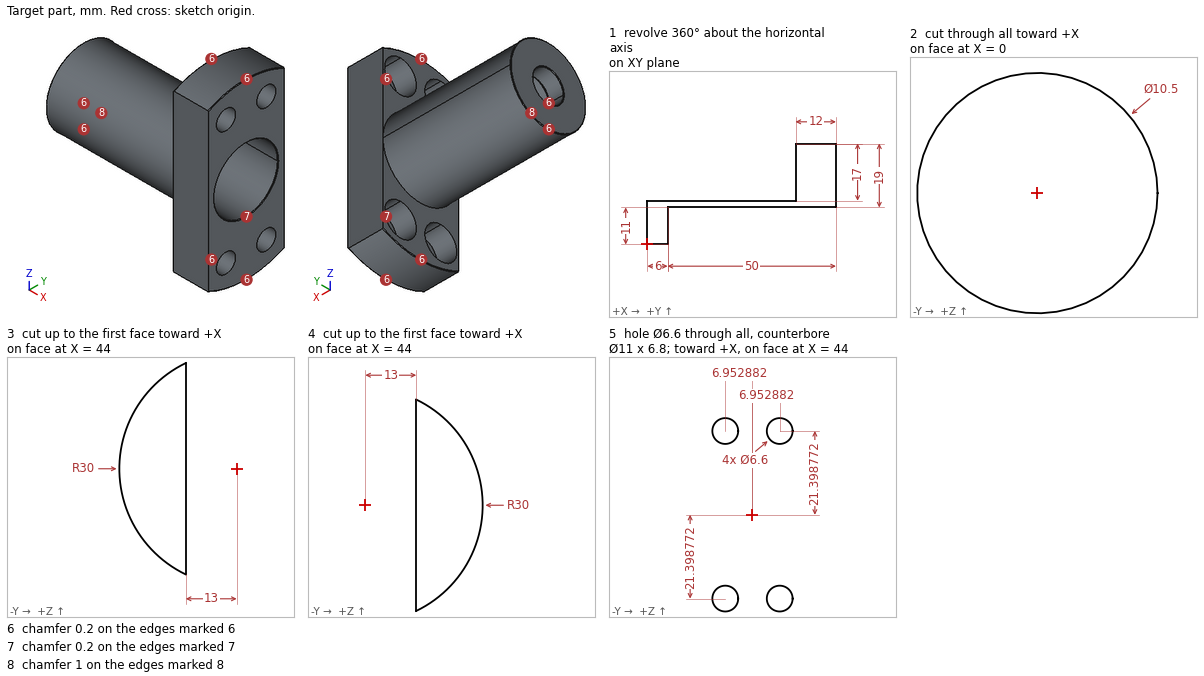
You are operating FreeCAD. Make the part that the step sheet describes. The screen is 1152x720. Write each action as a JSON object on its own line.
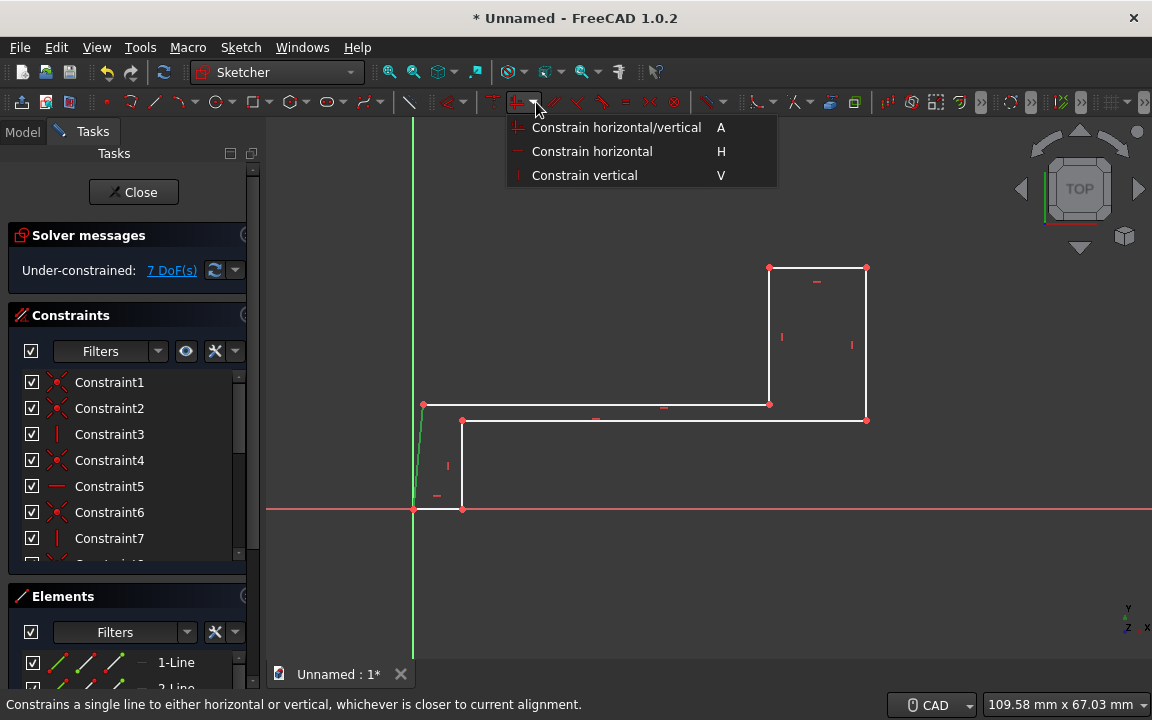
{"action": "left_click", "coordinate": [642, 175]}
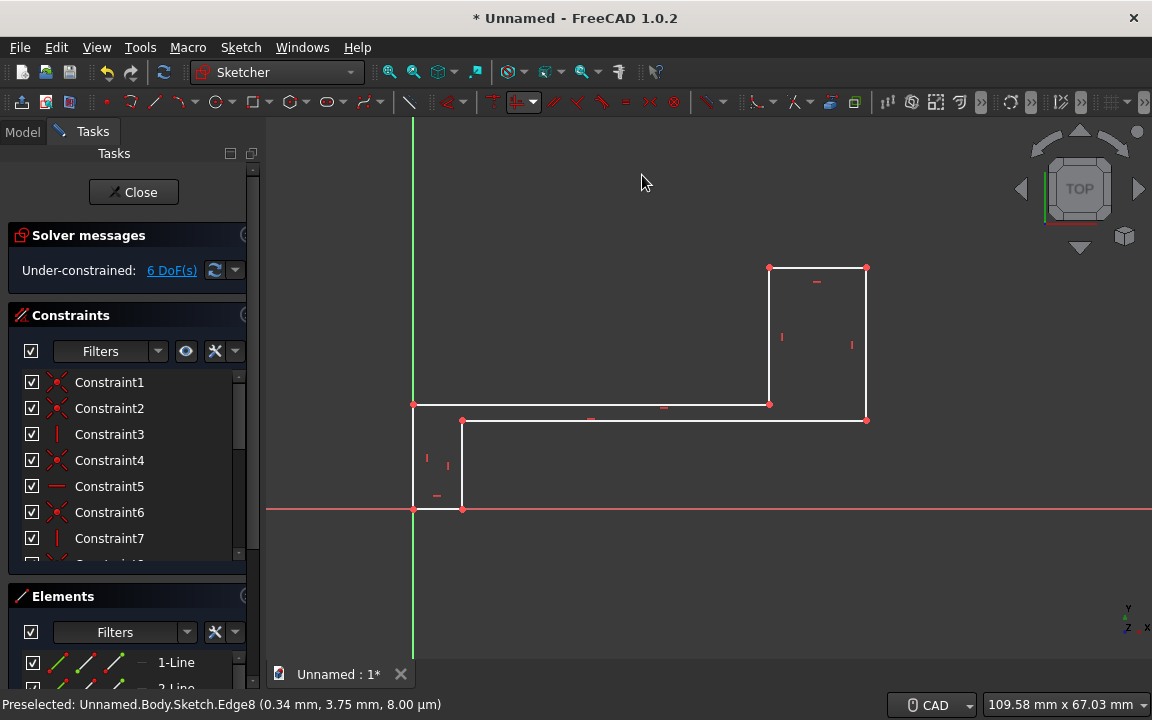
{"action": "left_click", "coordinate": [428, 509]}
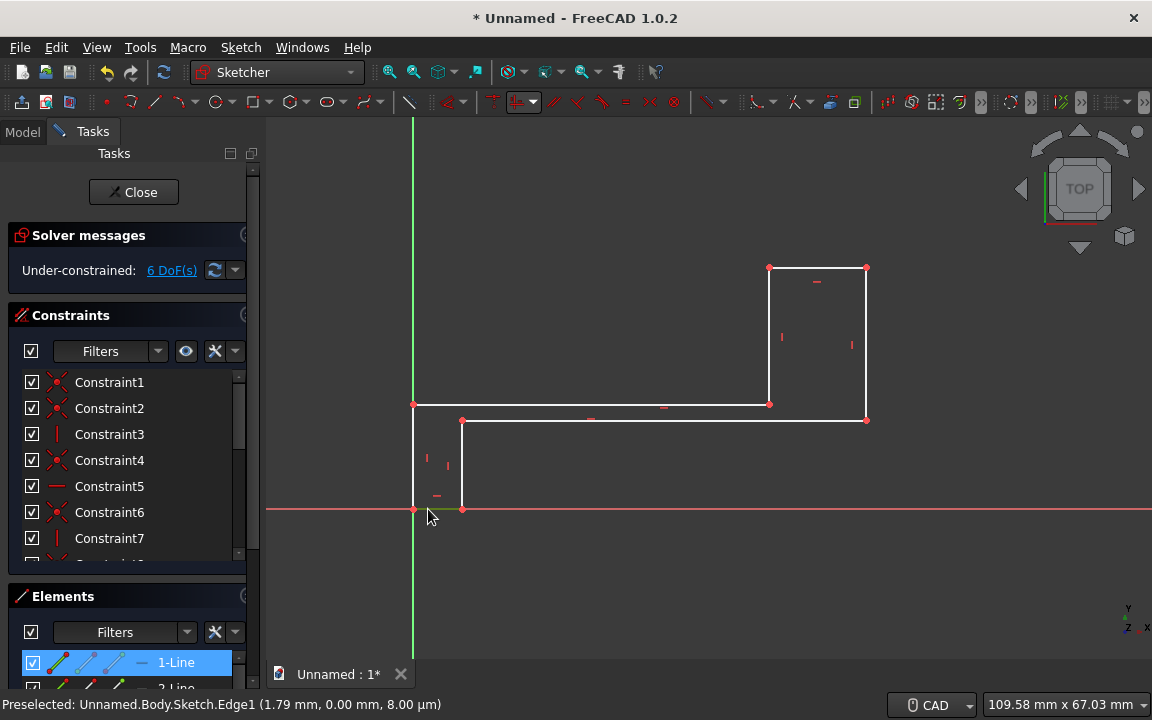
{"action": "key", "text": "l"}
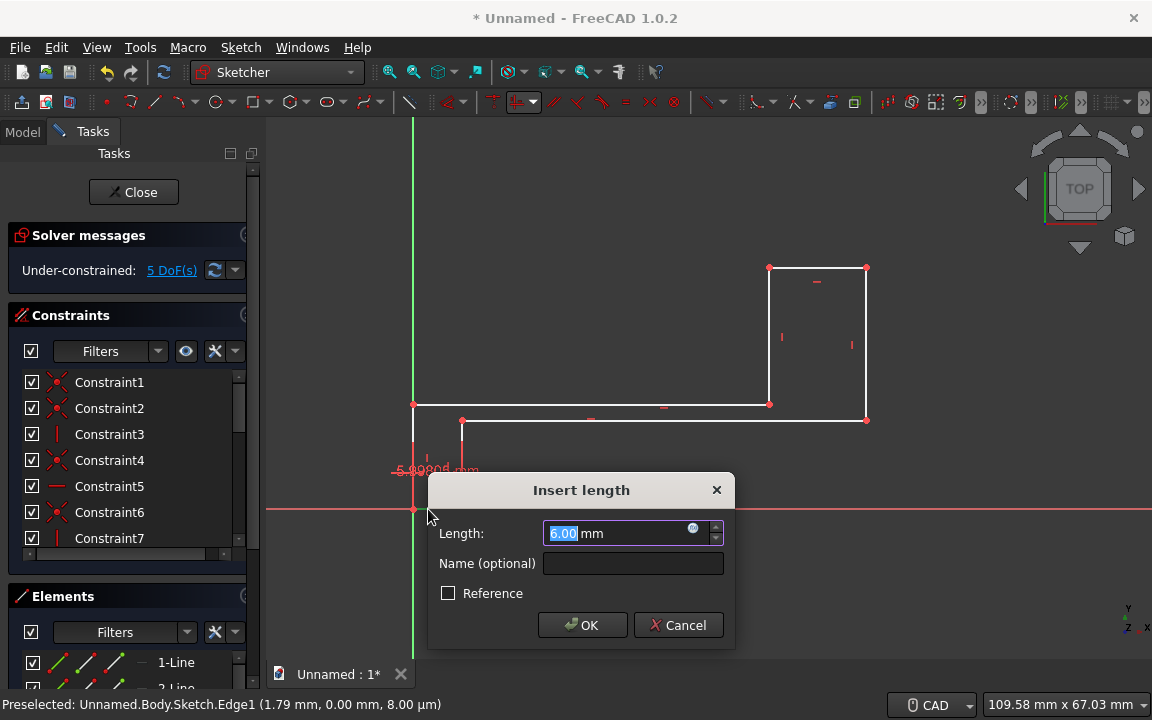
{"action": "type", "text": "6"}
{"action": "key", "text": "Return"}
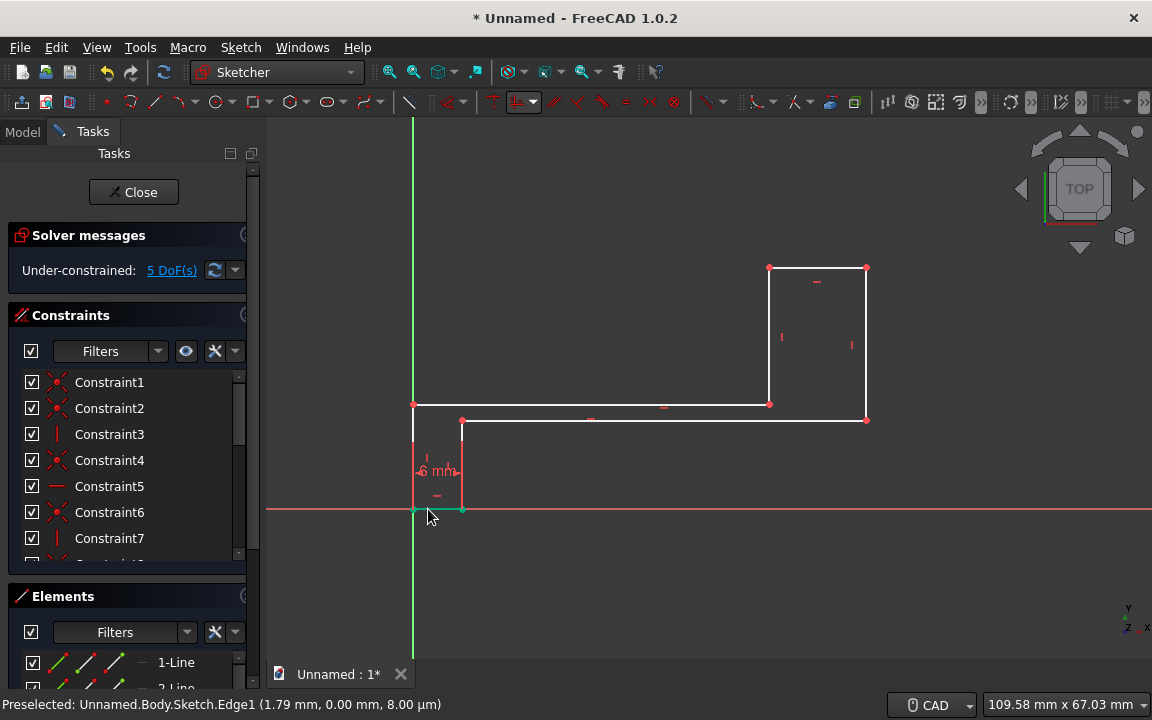
{"action": "left_click", "coordinate": [462, 483]}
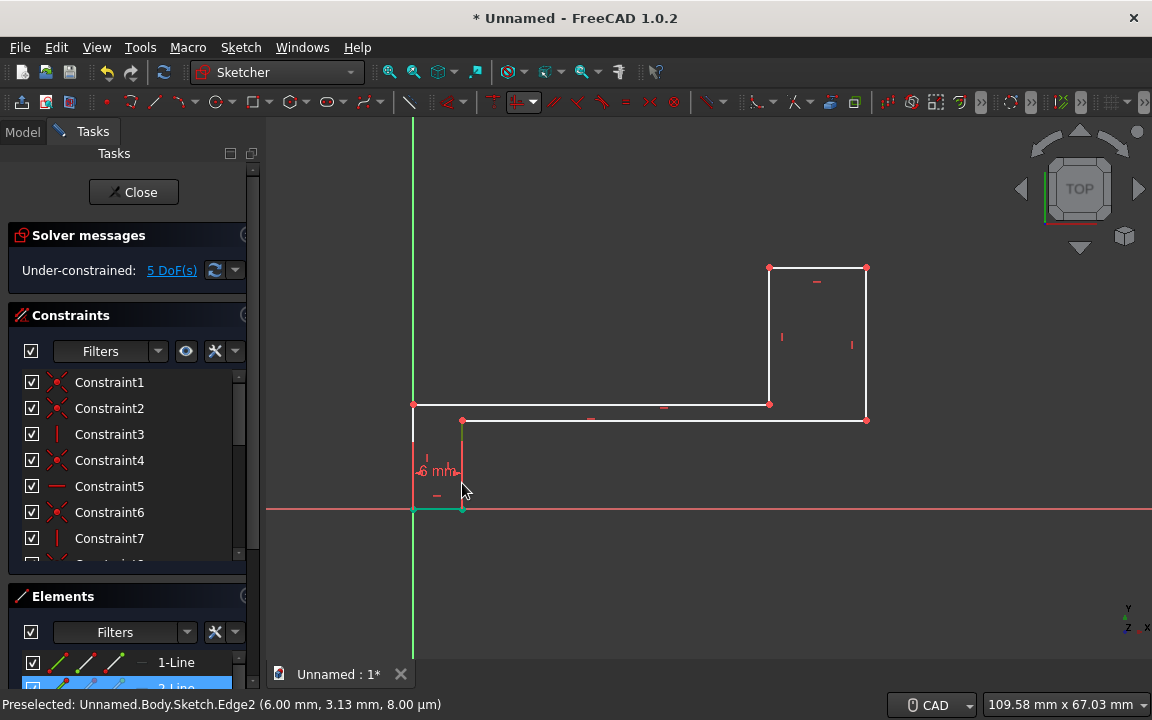
{"action": "key", "text": "i"}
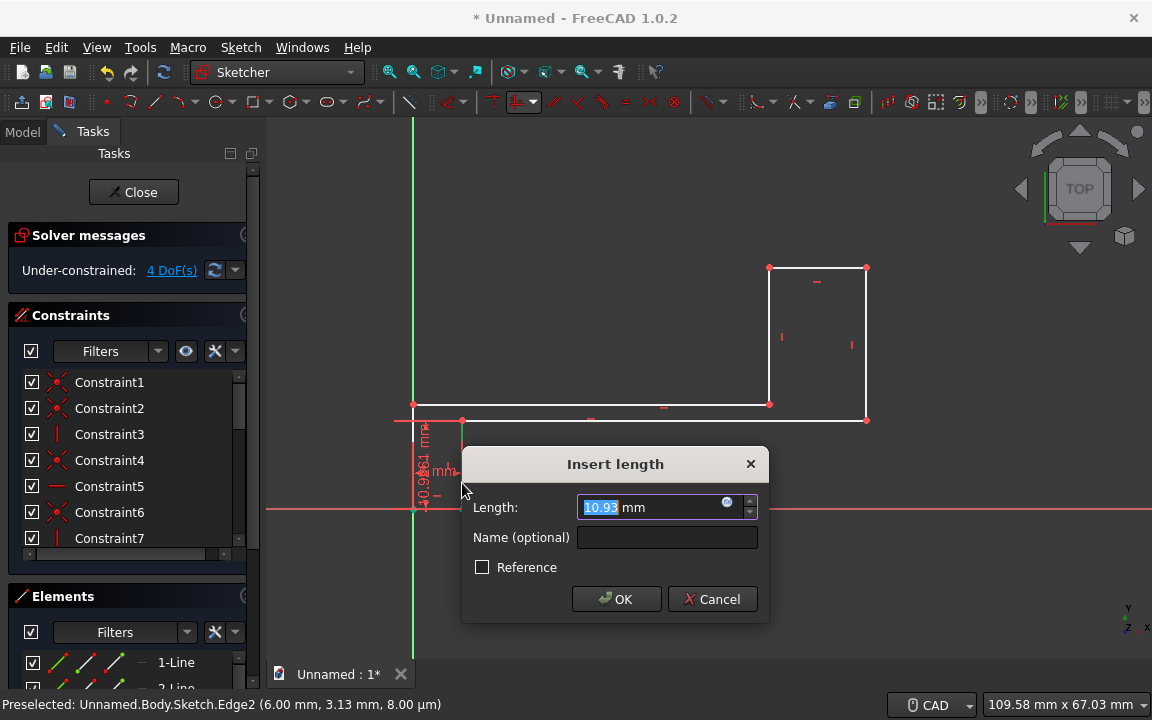
{"action": "type", "text": "11"}
{"action": "key", "text": "Return"}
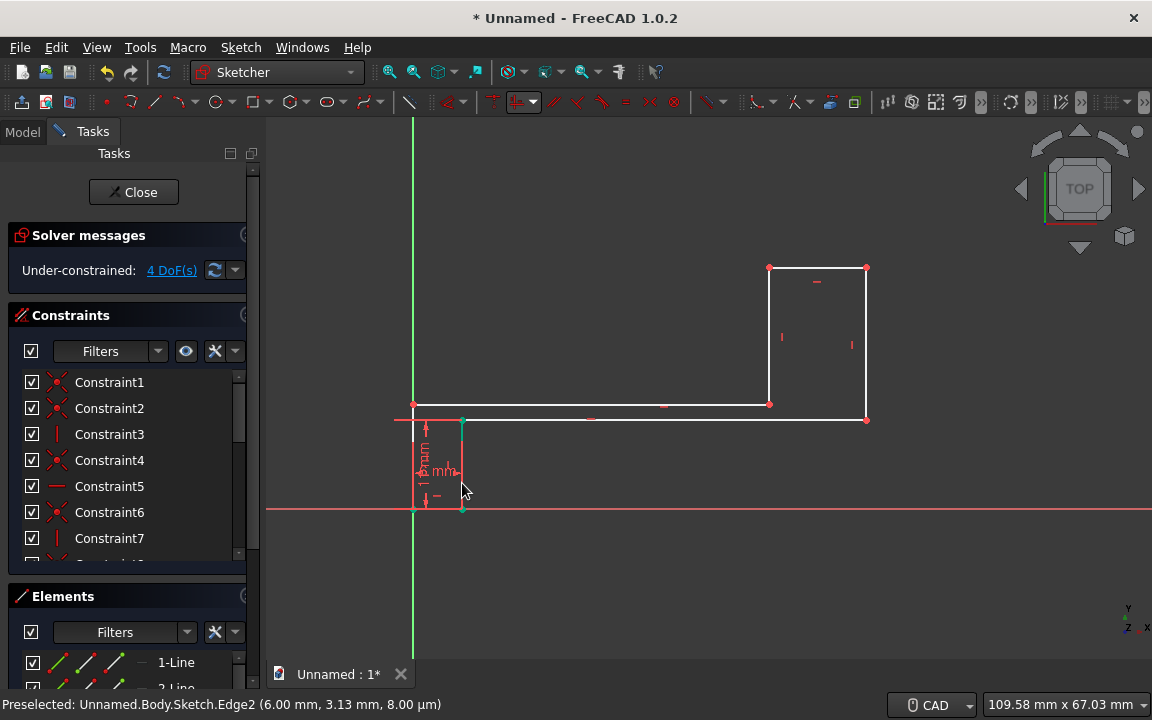
{"action": "left_click", "coordinate": [583, 420]}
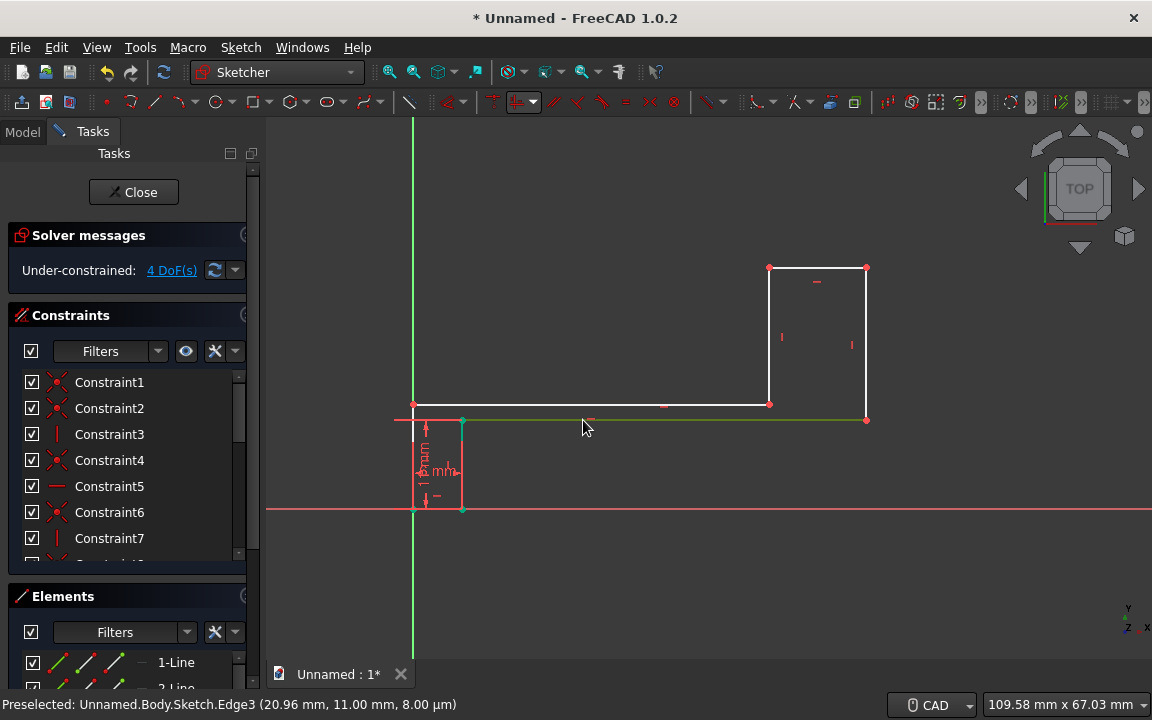
{"action": "key", "text": "l"}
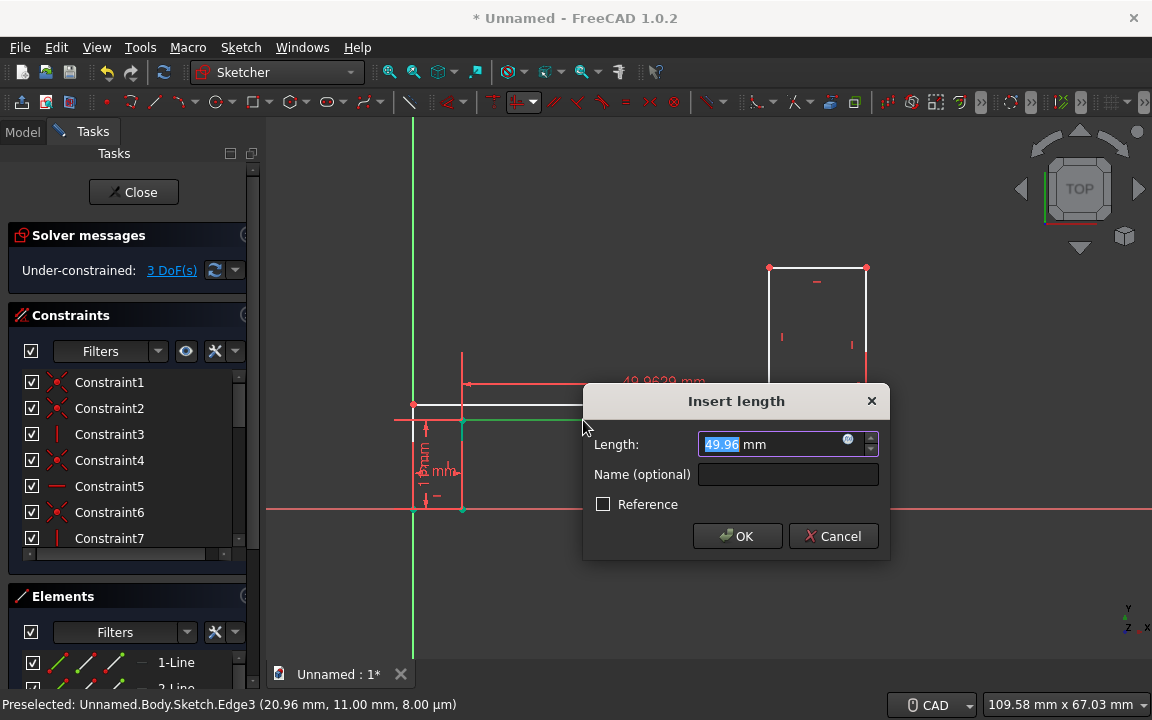
{"action": "type", "text": "50"}
{"action": "key", "text": "Return"}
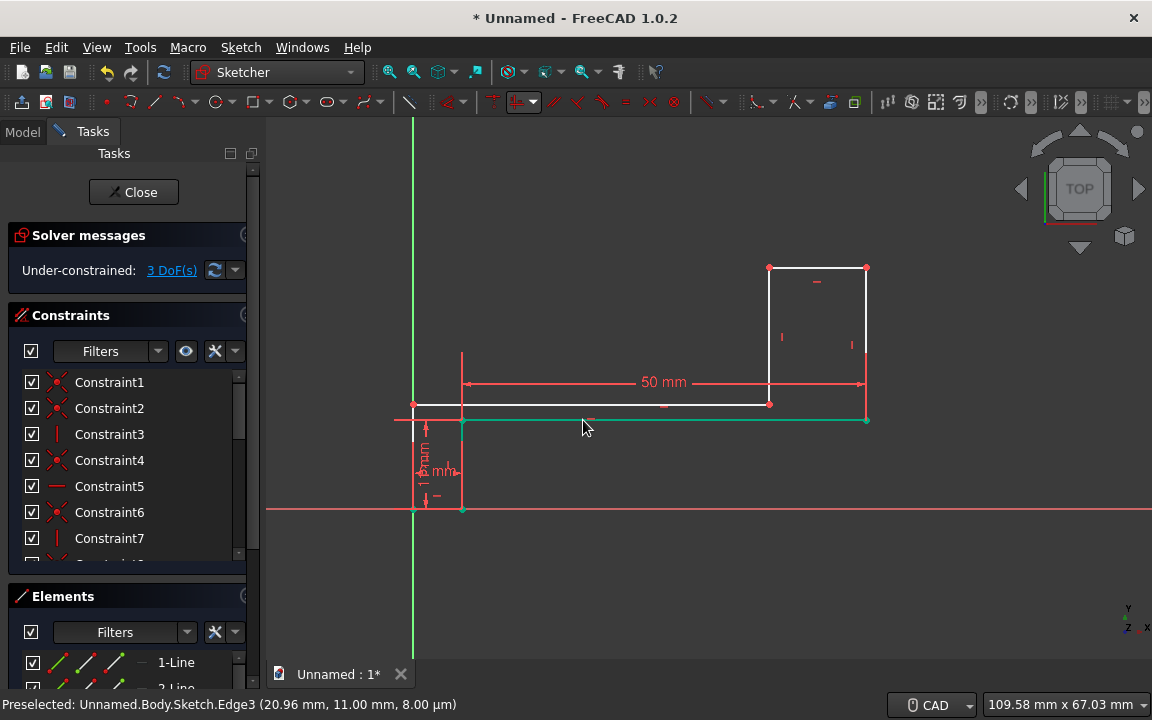
{"action": "left_click", "coordinate": [866, 375]}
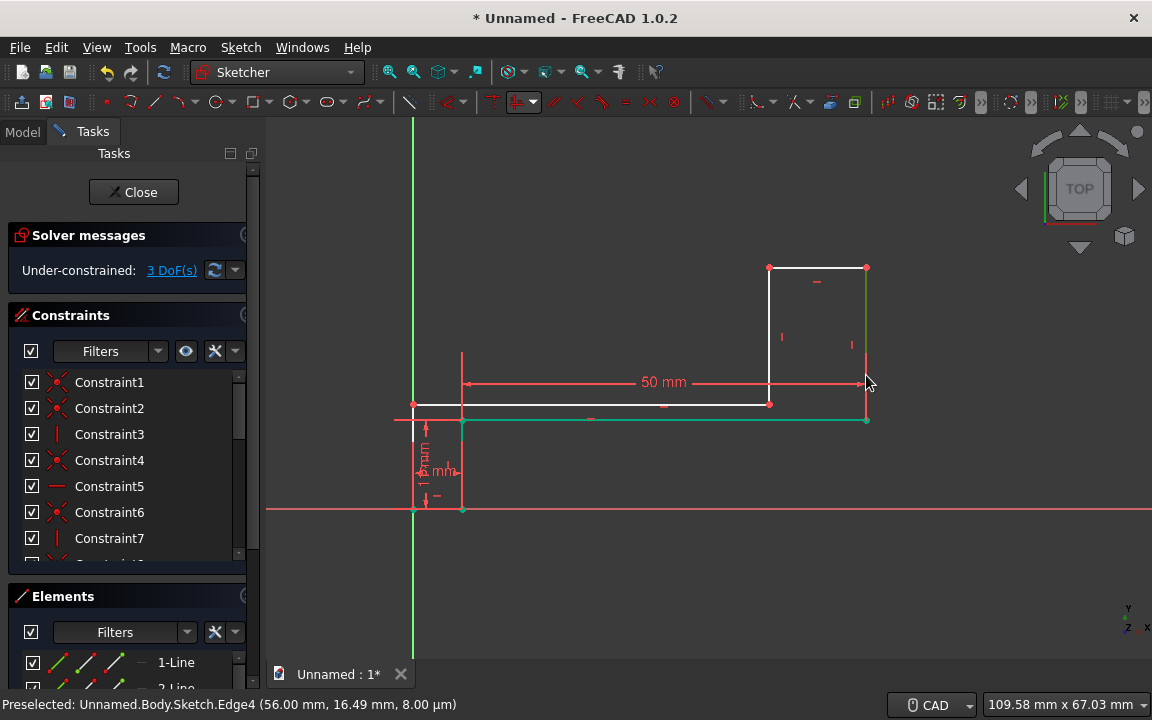
{"action": "key", "text": "i"}